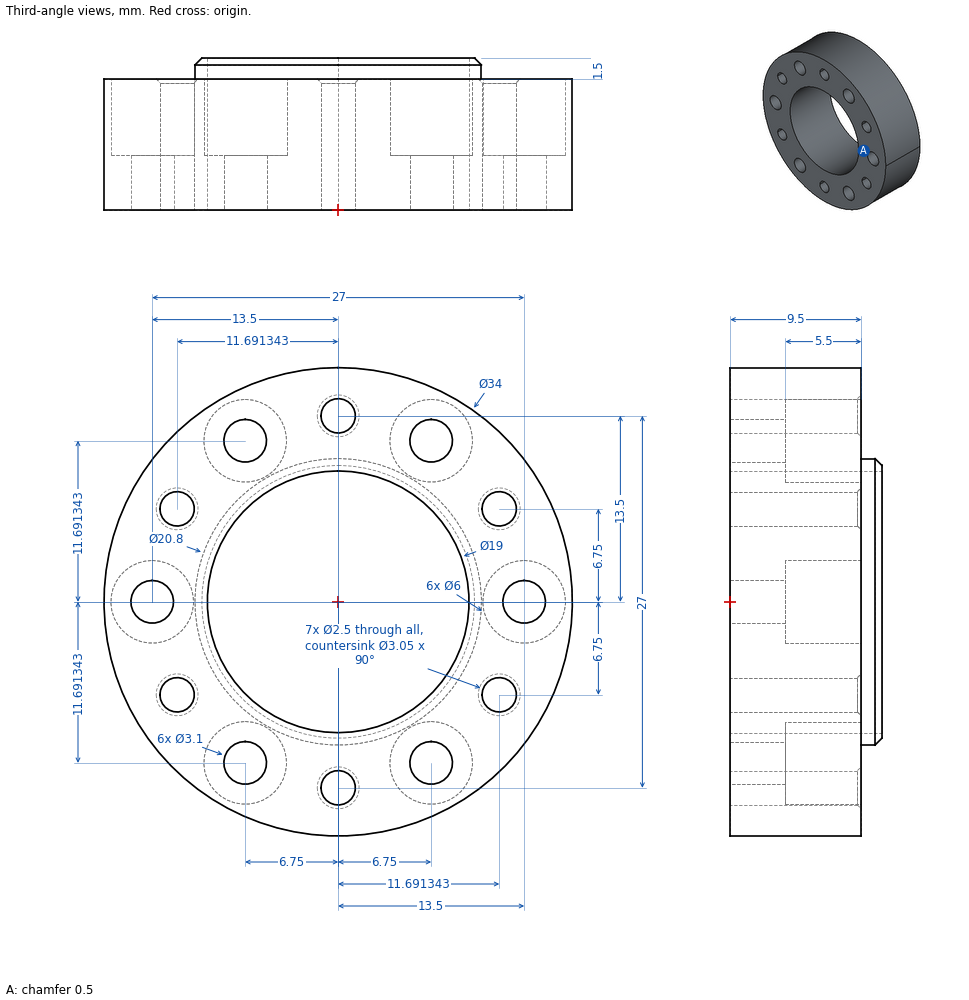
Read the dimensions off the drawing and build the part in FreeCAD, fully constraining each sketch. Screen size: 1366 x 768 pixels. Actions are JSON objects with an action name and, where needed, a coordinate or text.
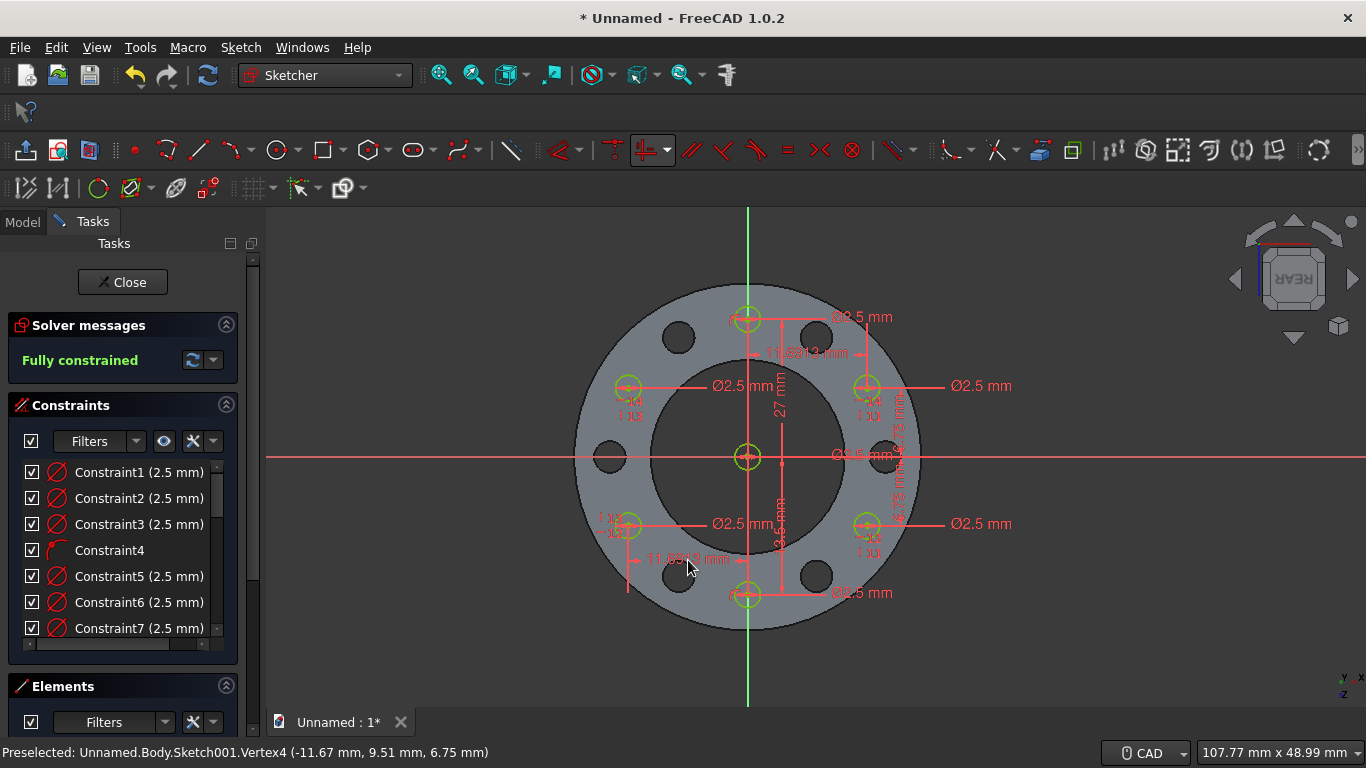
{"action": "left_click", "coordinate": [123, 282]}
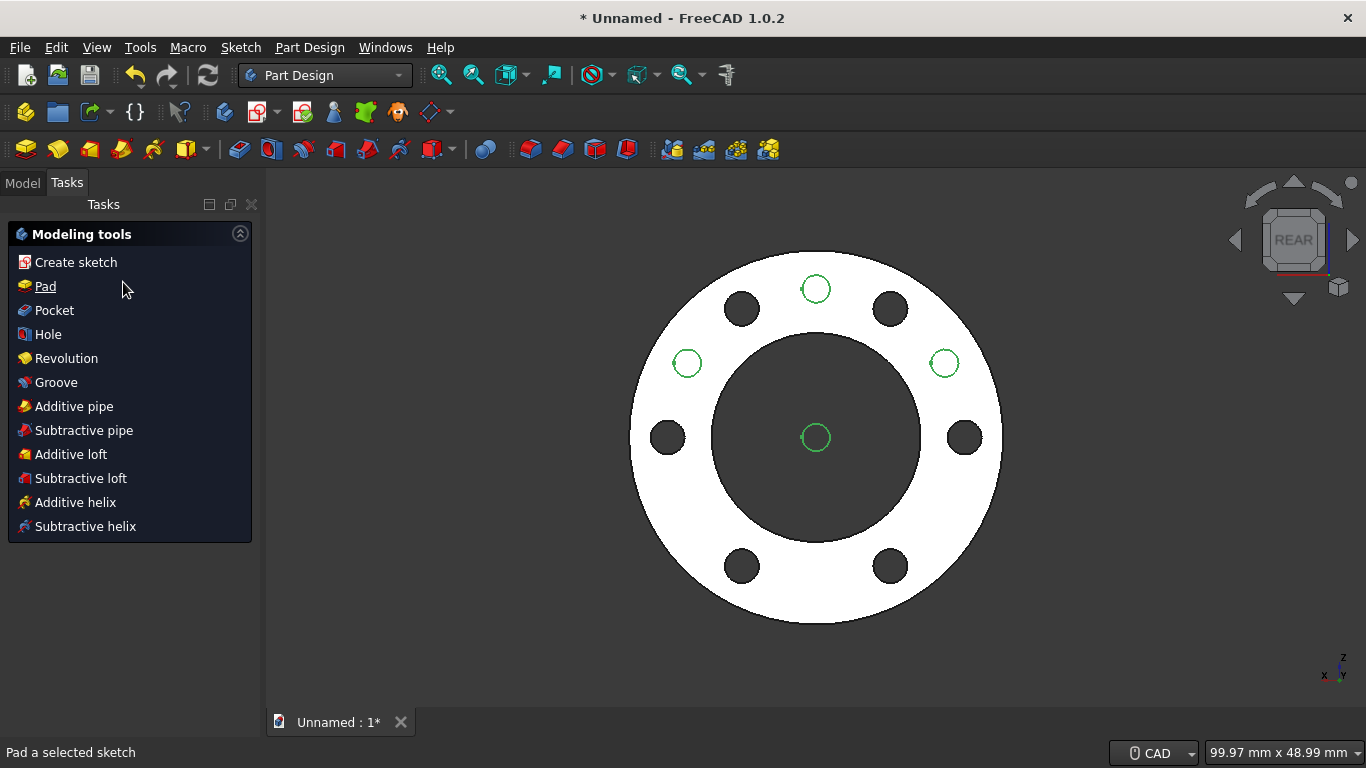
{"action": "left_click", "coordinate": [272, 150]}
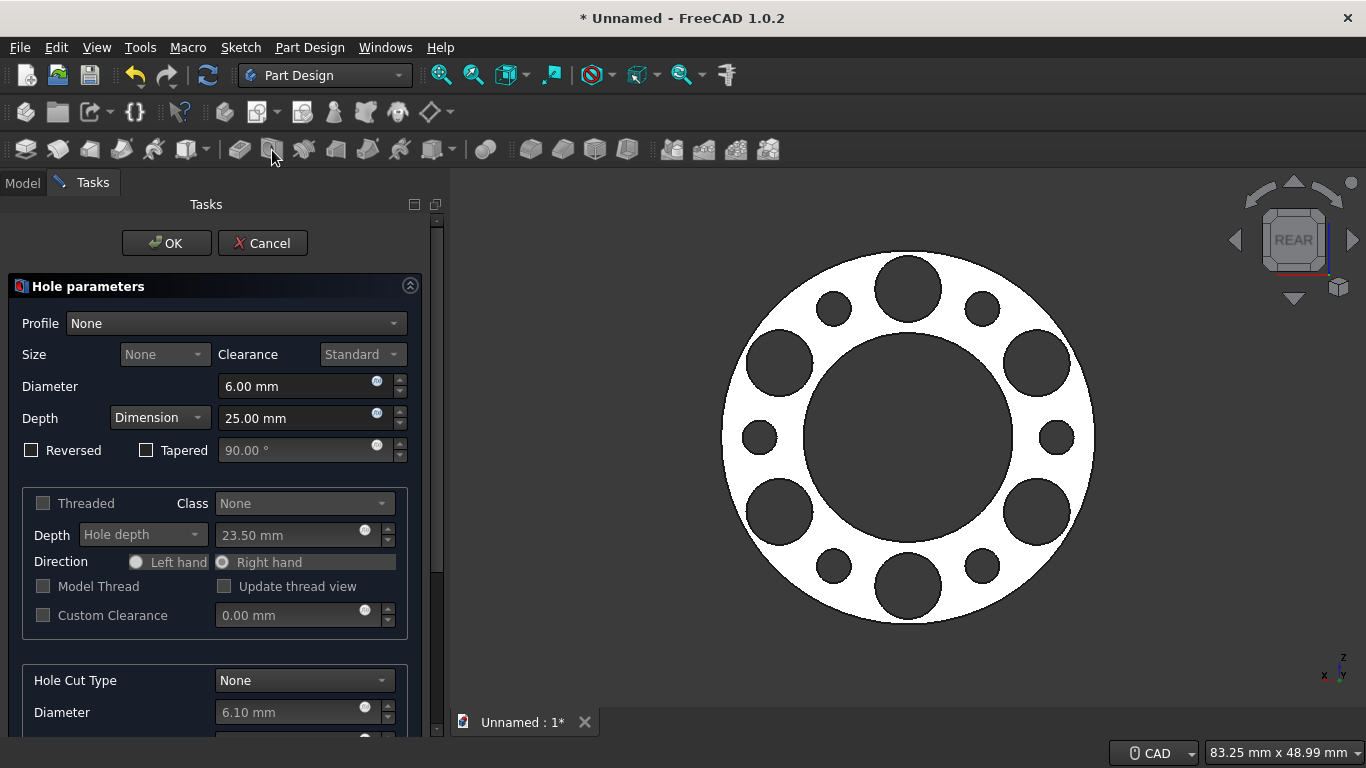
{"action": "triple_click", "coordinate": [305, 386]}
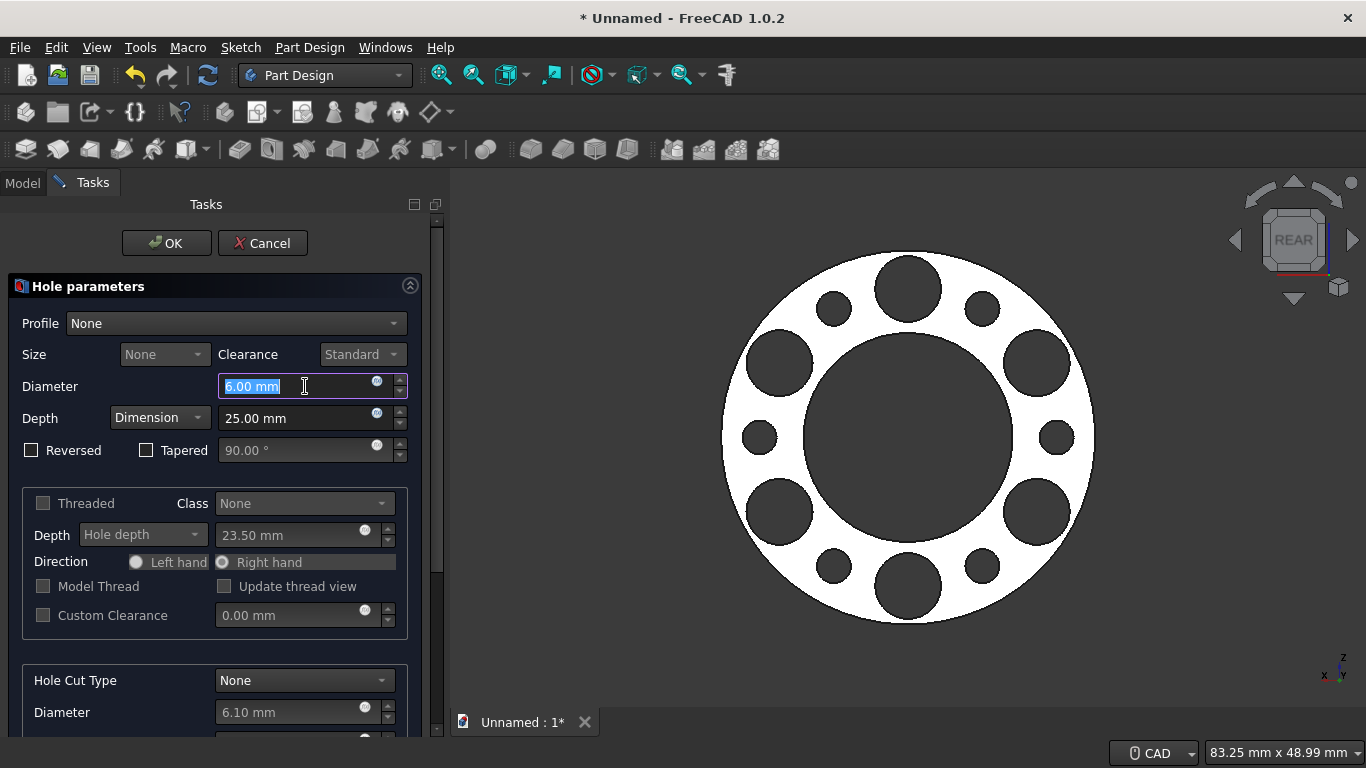
{"action": "type", "text": "2.5"}
{"action": "key", "text": "Tab"}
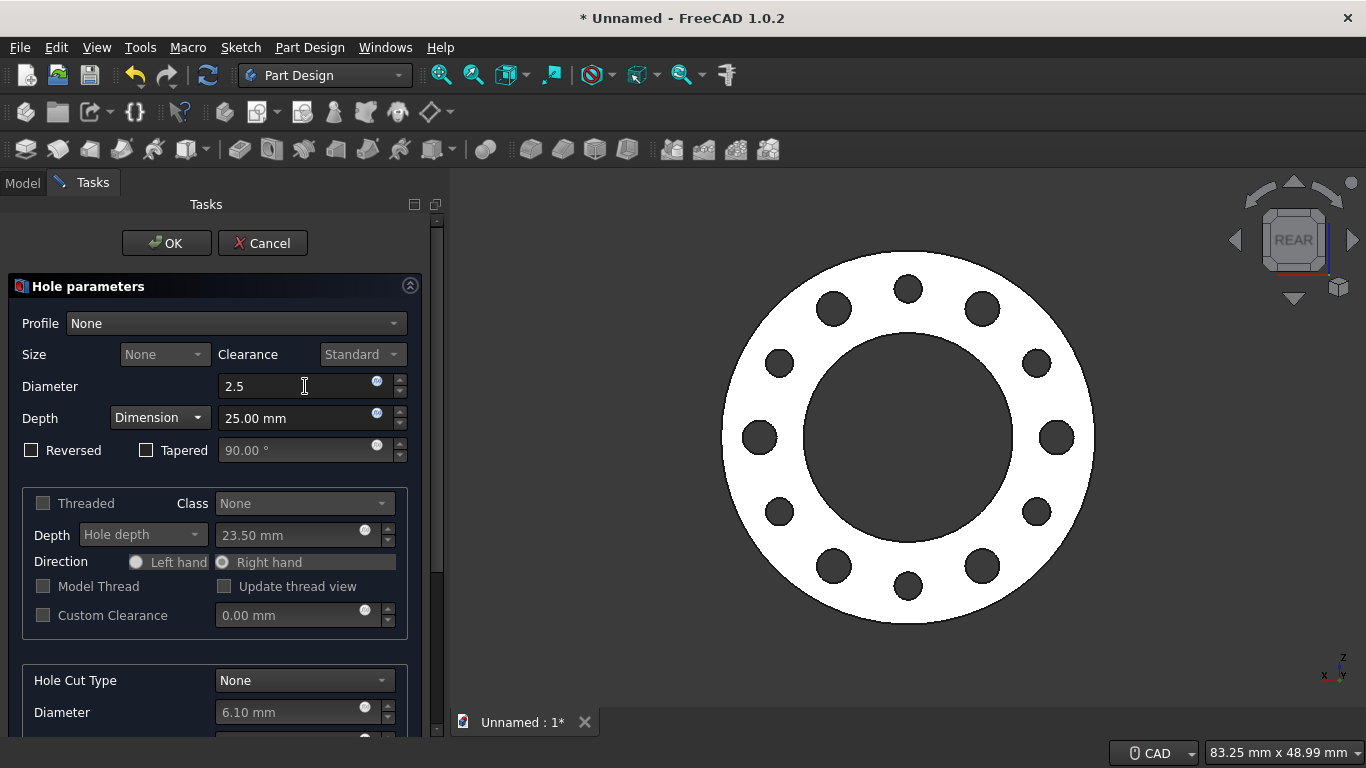
{"action": "left_click", "coordinate": [161, 418]}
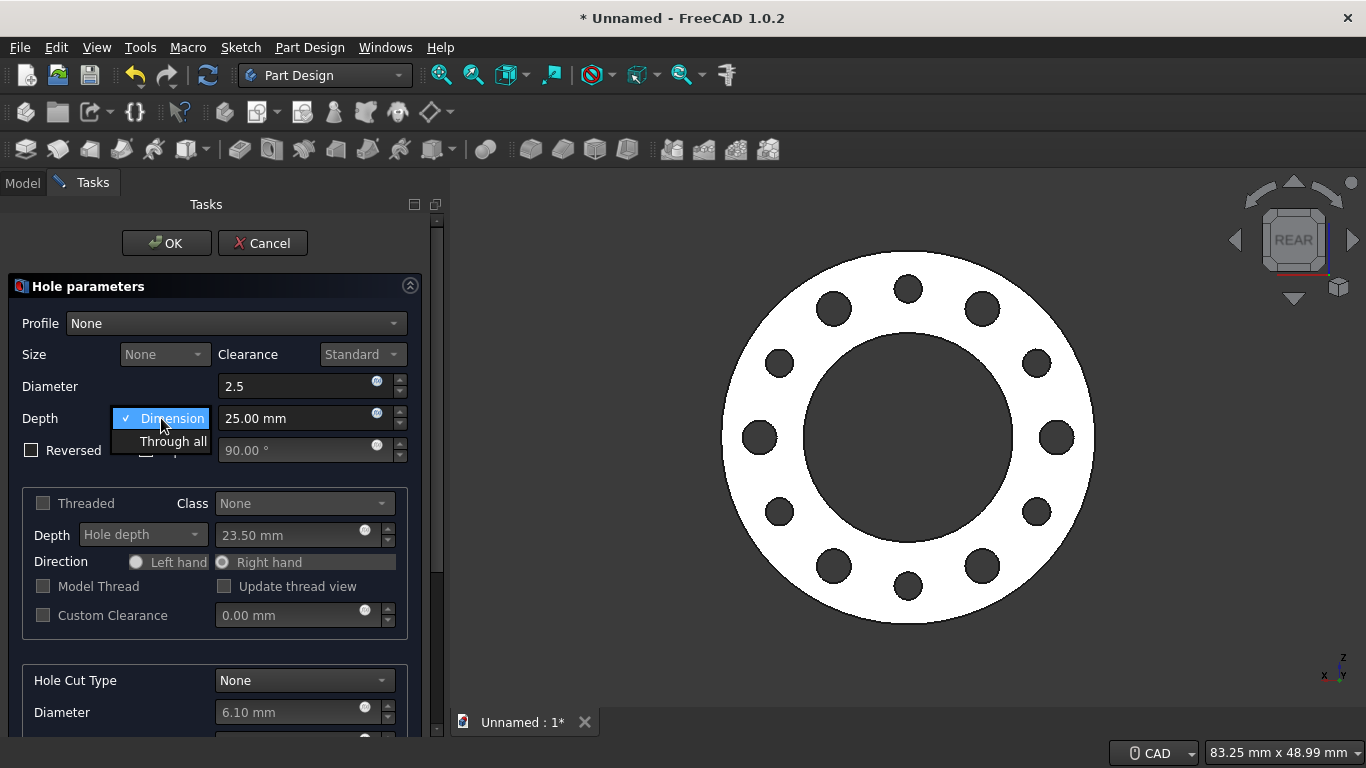
{"action": "left_click", "coordinate": [160, 442]}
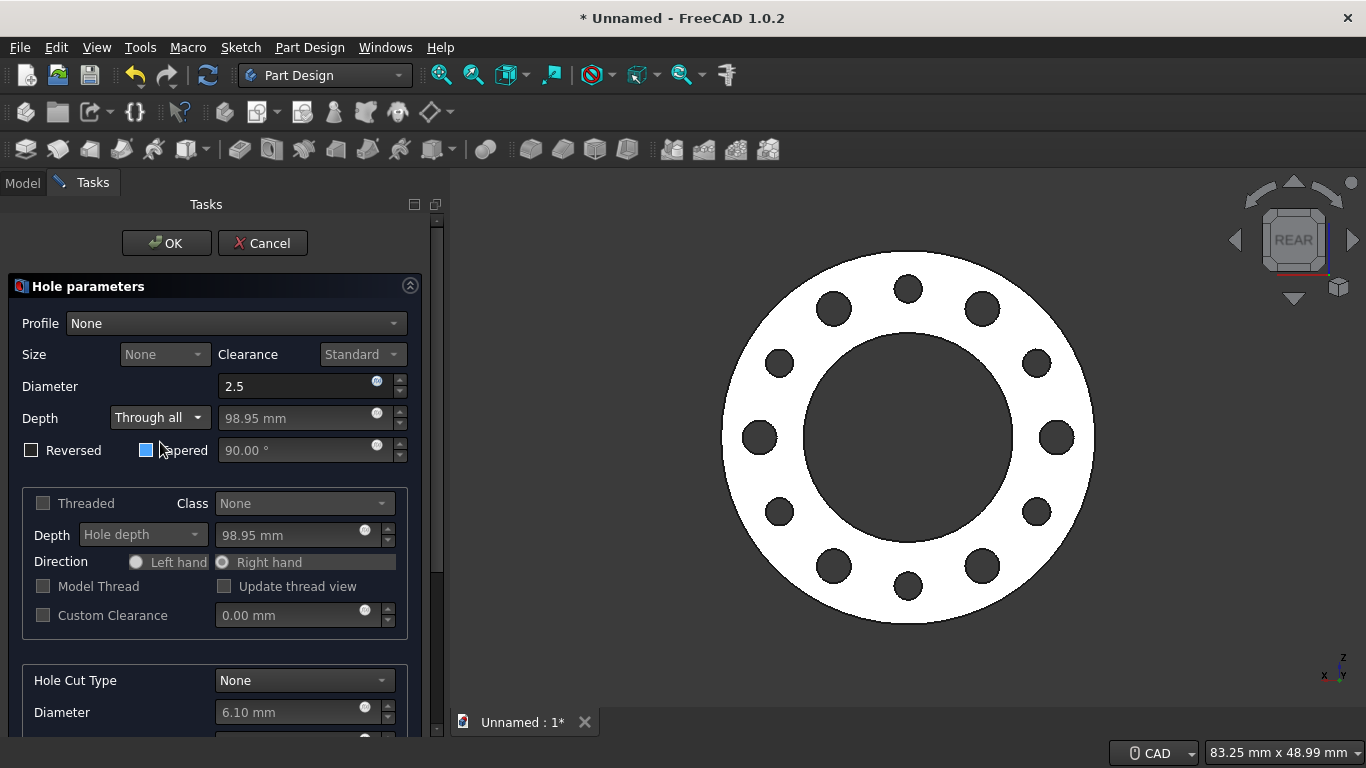
{"action": "left_click", "coordinate": [306, 680]}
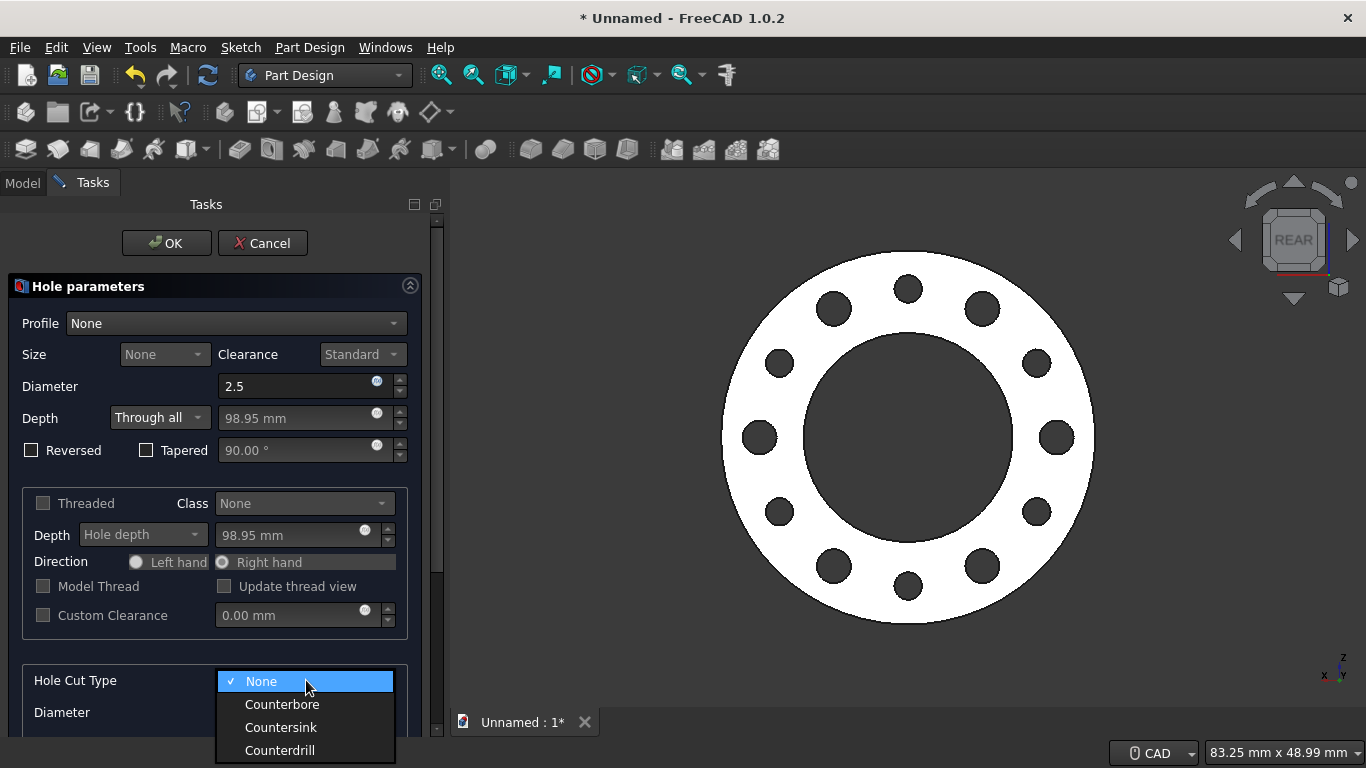
{"action": "left_click", "coordinate": [304, 728]}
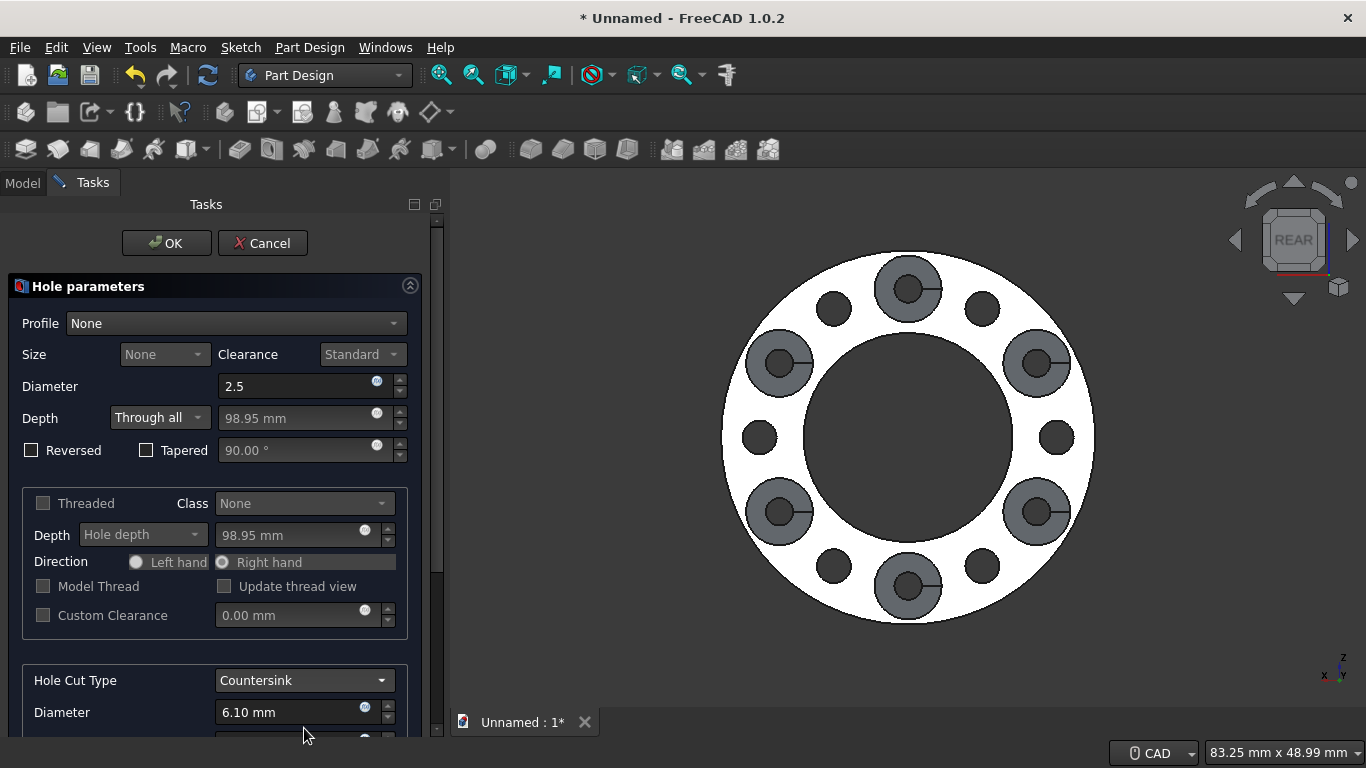
{"action": "triple_click", "coordinate": [298, 712]}